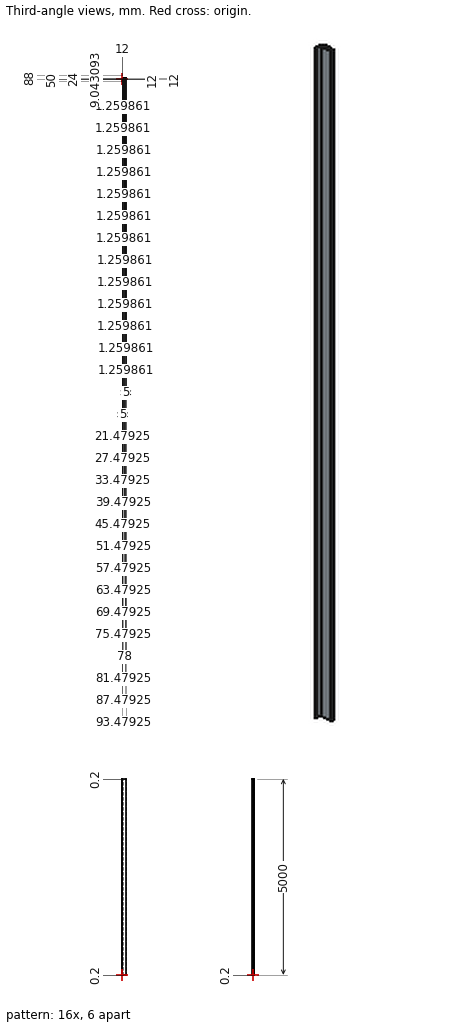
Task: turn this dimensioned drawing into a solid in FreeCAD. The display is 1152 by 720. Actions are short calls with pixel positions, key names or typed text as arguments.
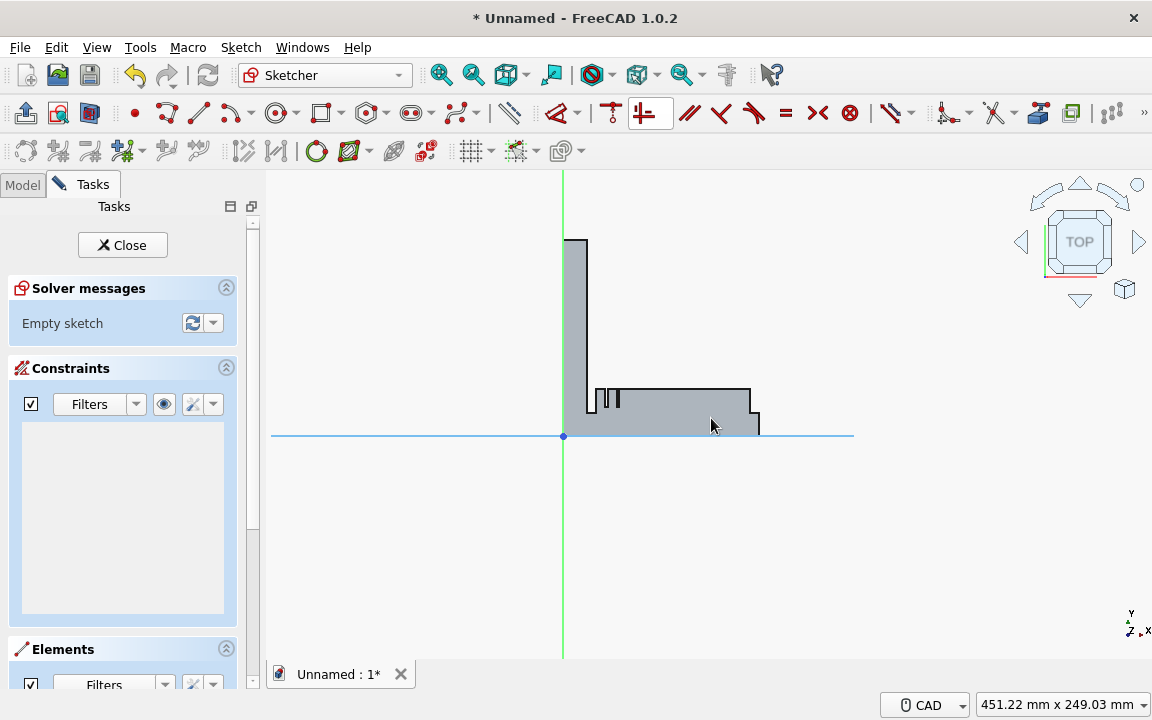
scroll(629, 397, up, 14)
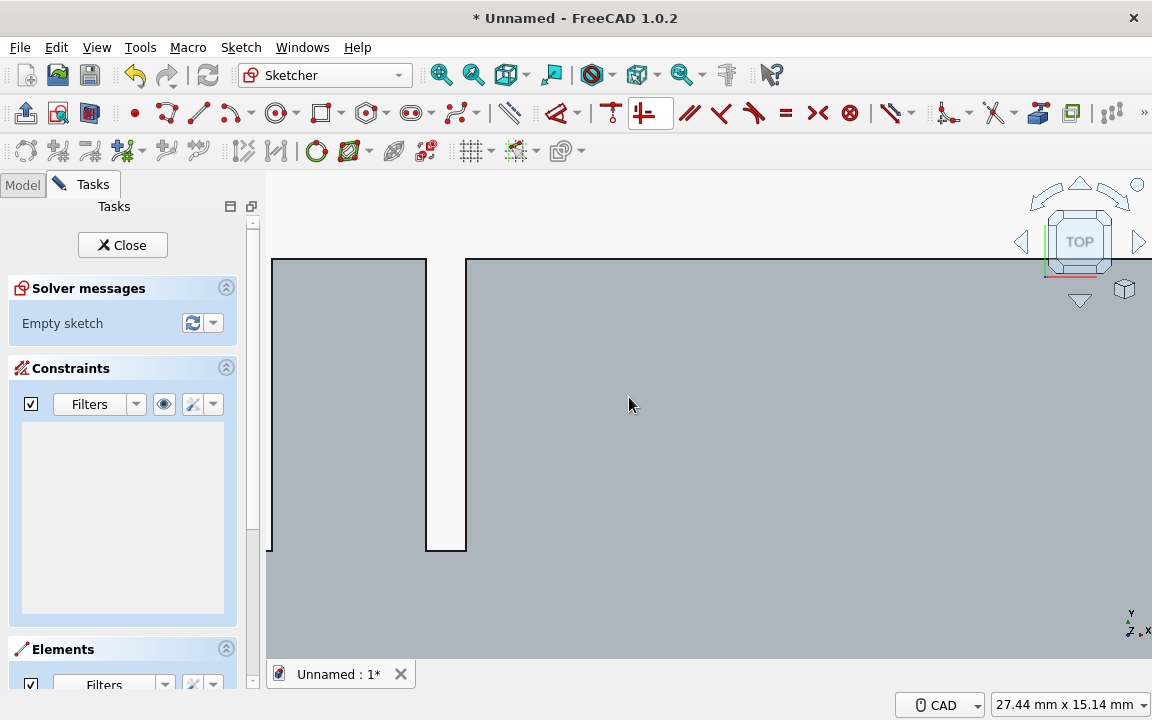
click(322, 114)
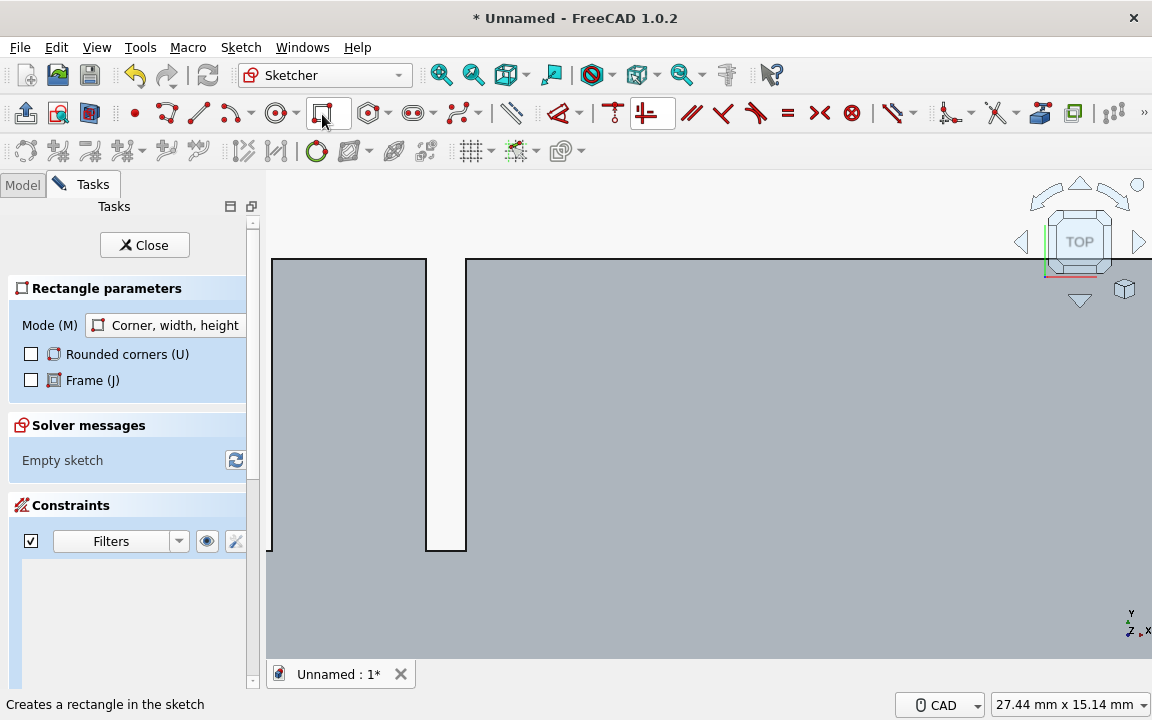
click(619, 259)
click(660, 551)
key(Escape)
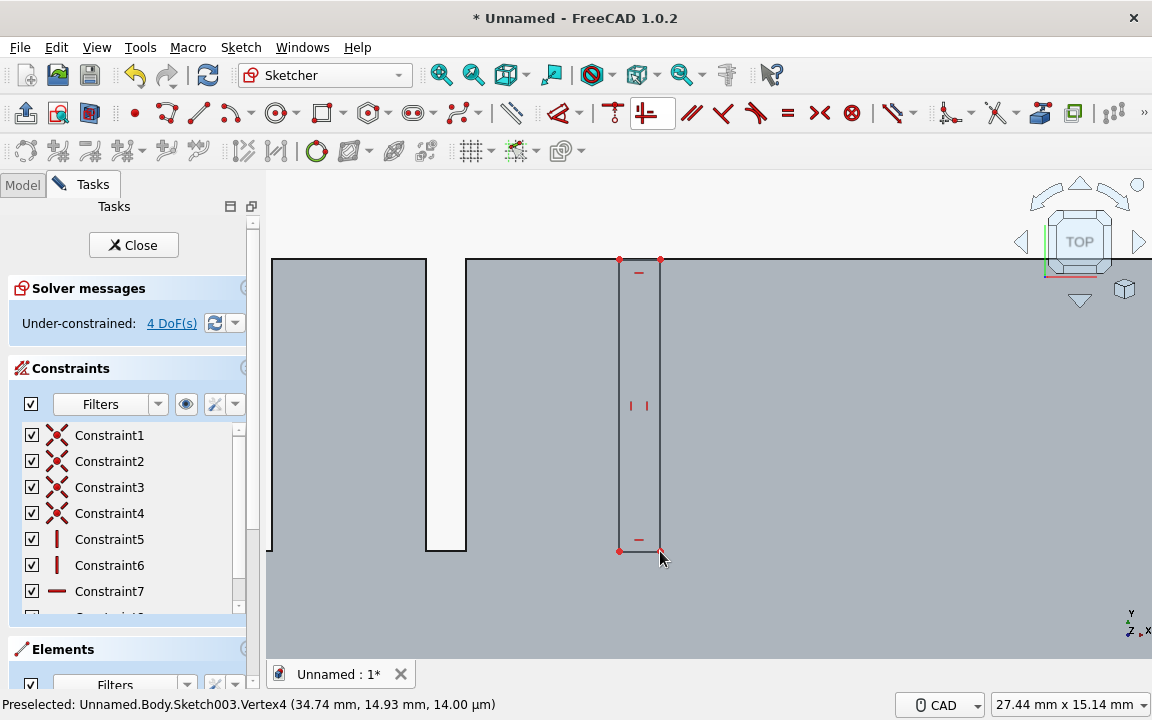
key(d)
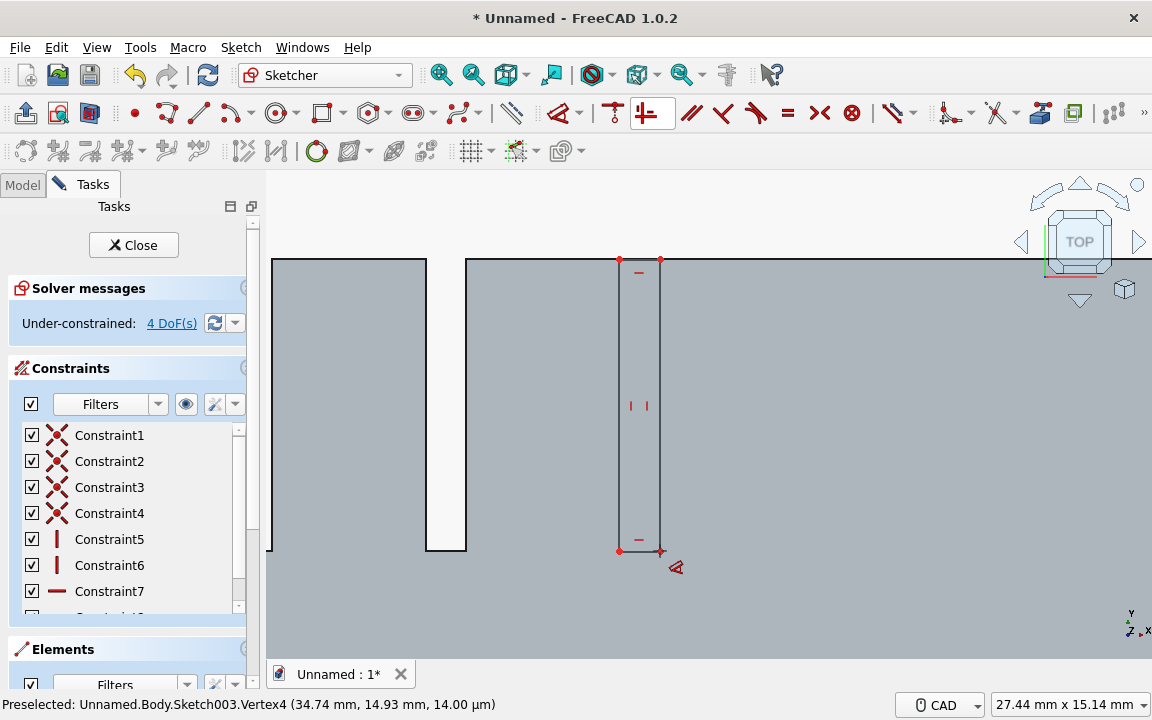
click(619, 260)
click(653, 575)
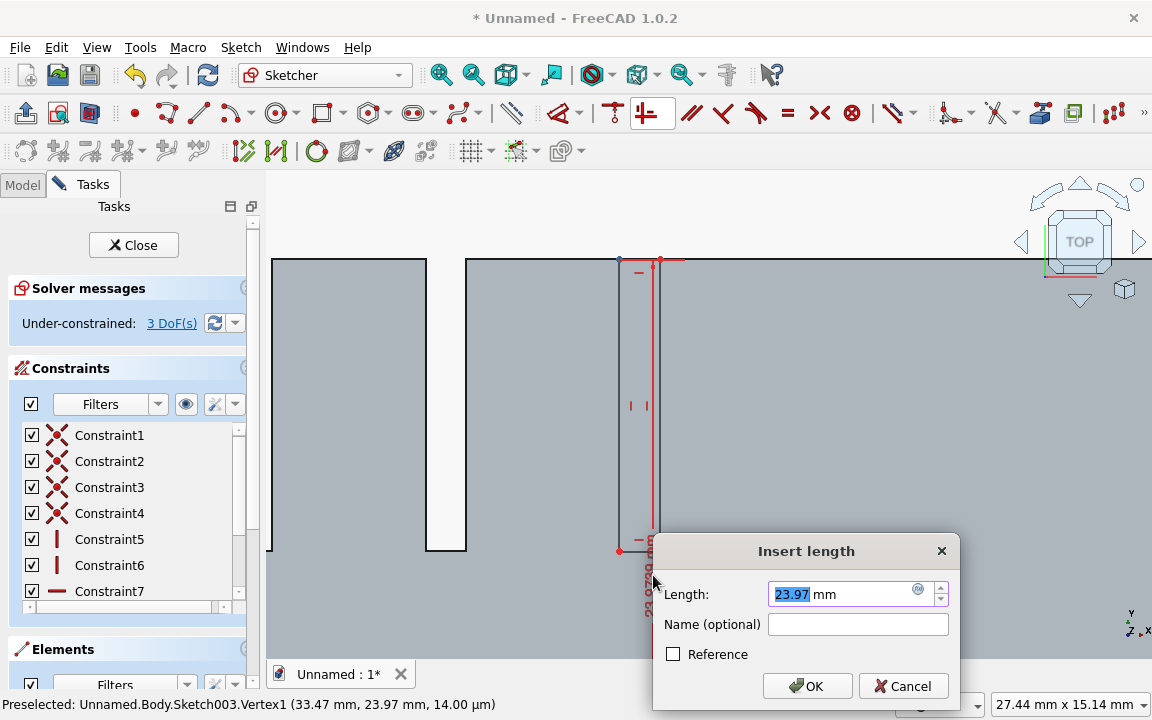
text(24)
key(Return)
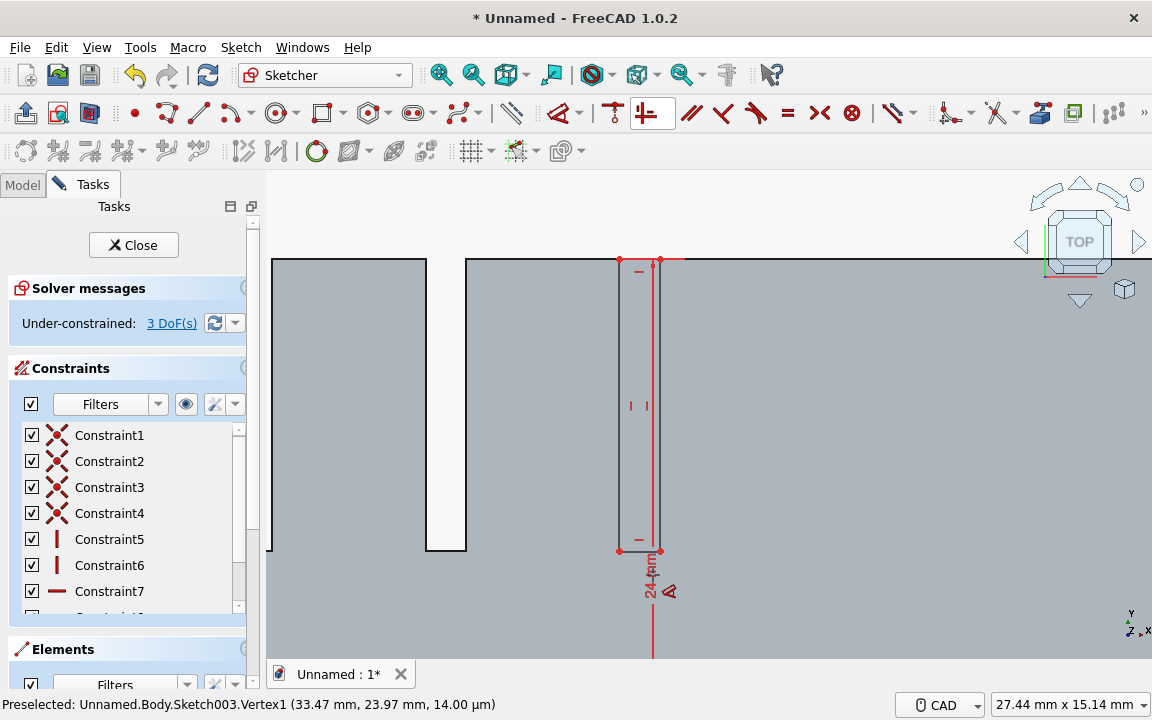
click(619, 347)
click(585, 406)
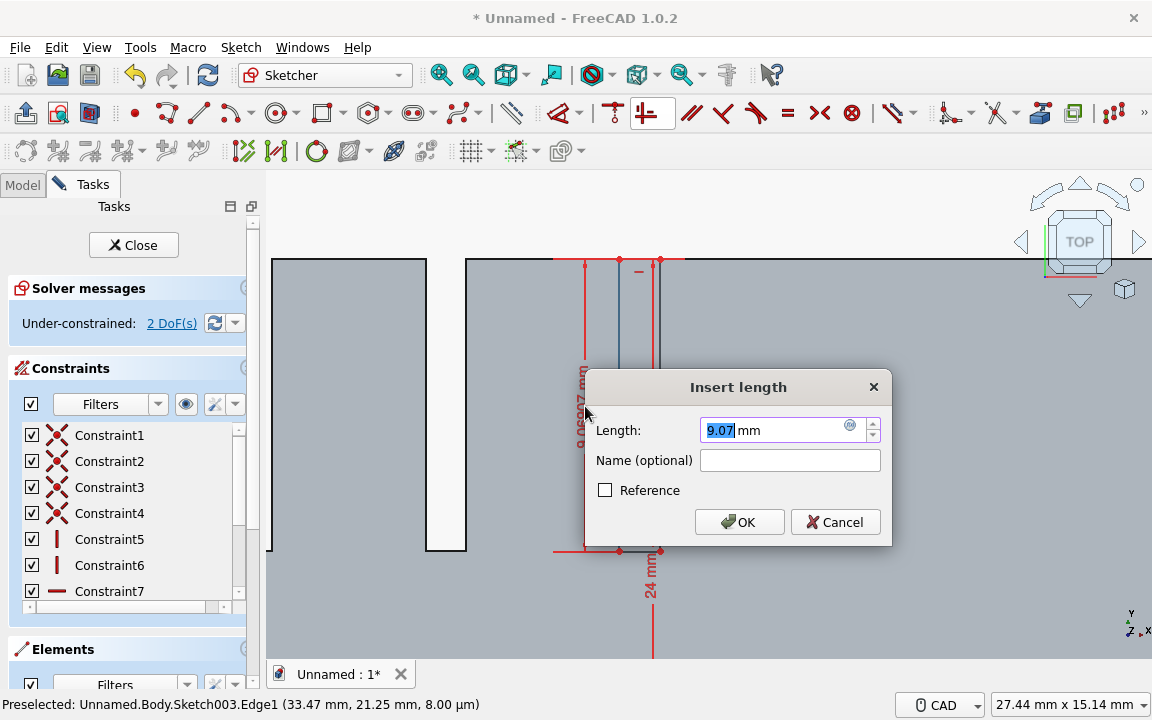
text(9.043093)
key(Return)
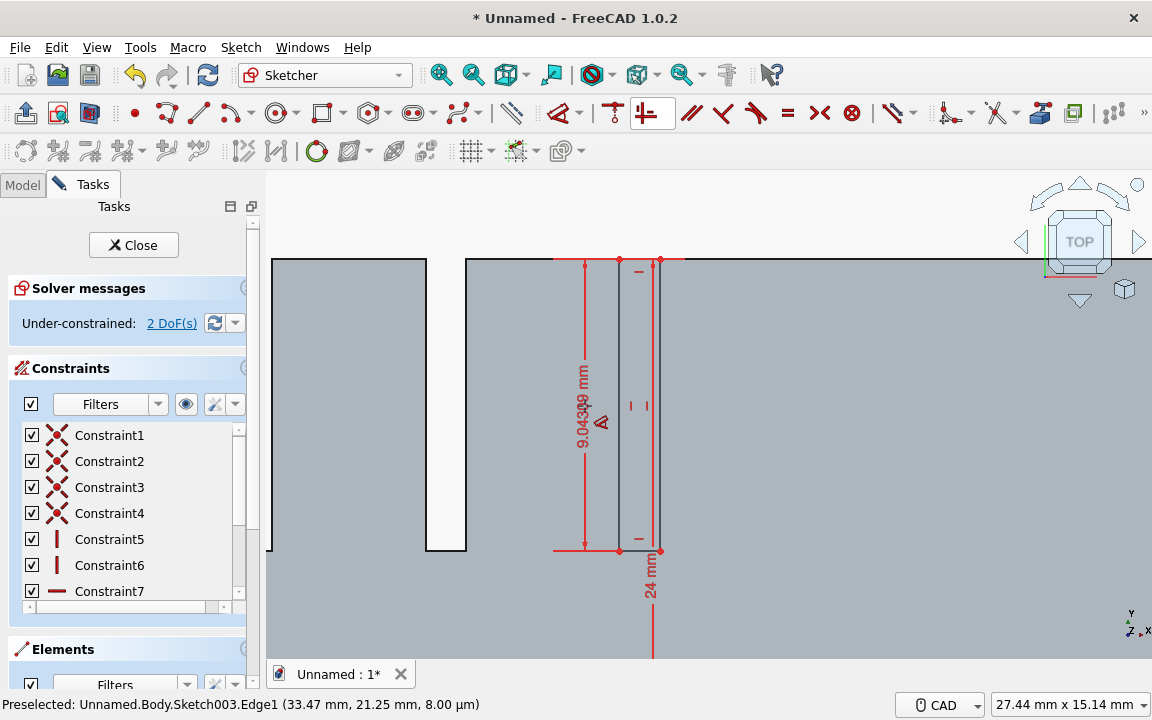
click(631, 551)
click(640, 517)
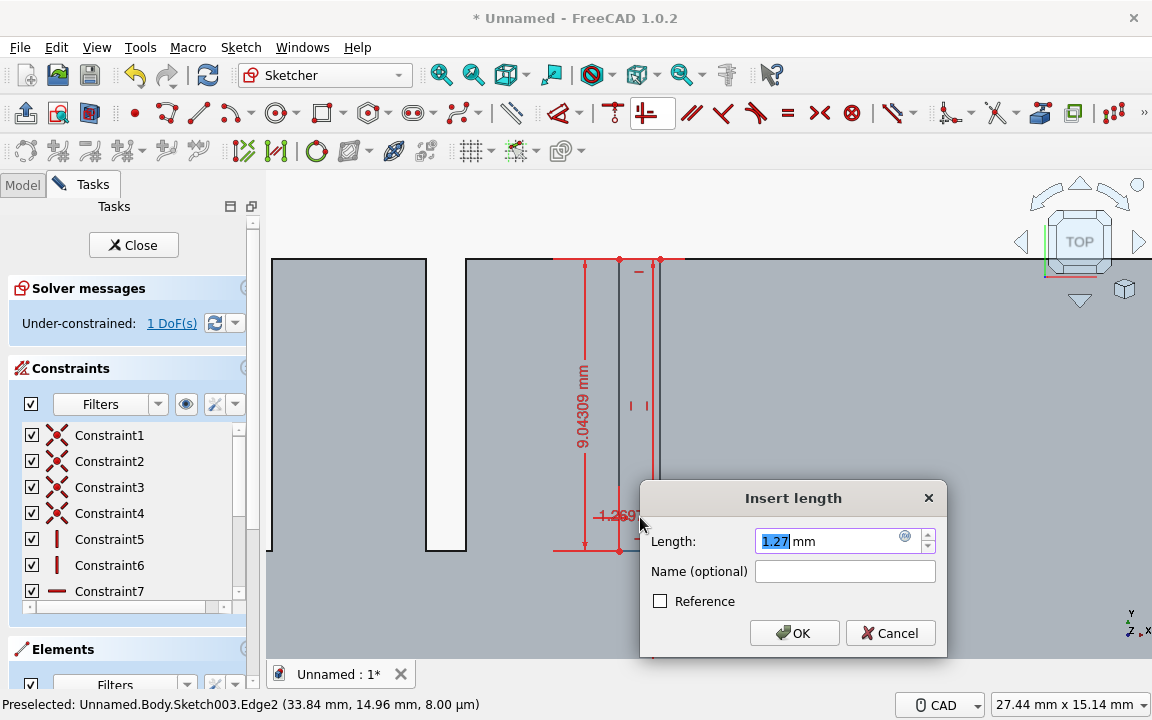
text(1.259861)
key(Return)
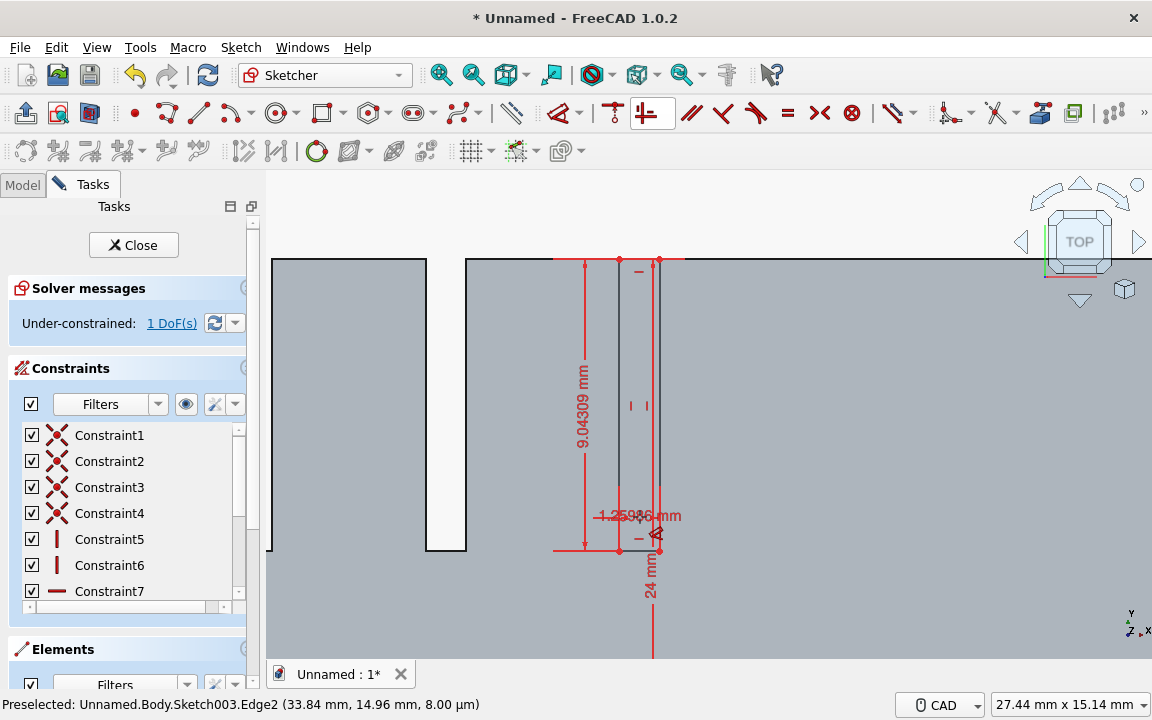
click(619, 259)
click(457, 225)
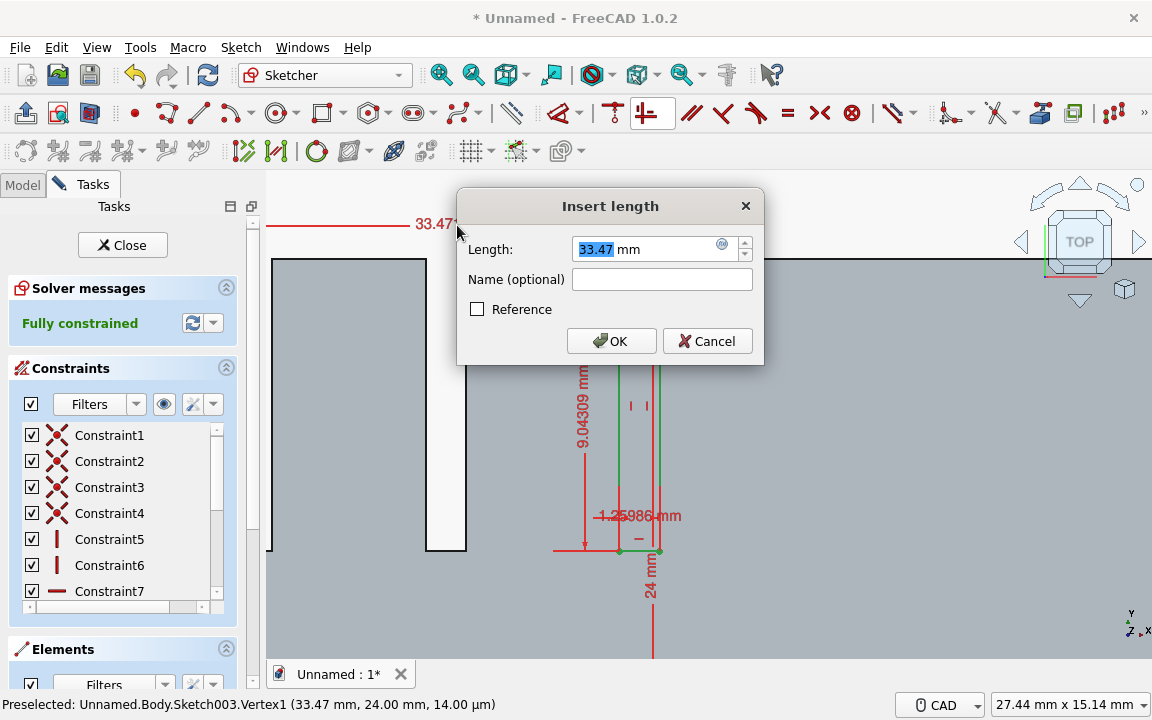
text(33.47925)
key(Return)
key(Escape)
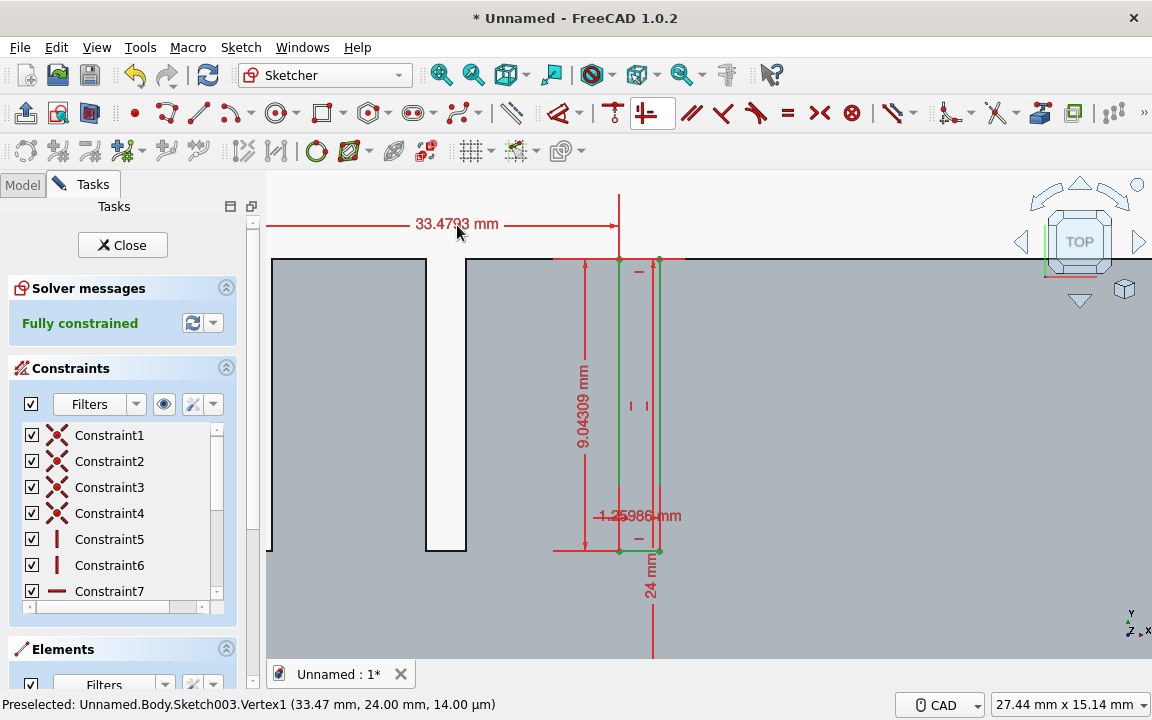
click(123, 245)